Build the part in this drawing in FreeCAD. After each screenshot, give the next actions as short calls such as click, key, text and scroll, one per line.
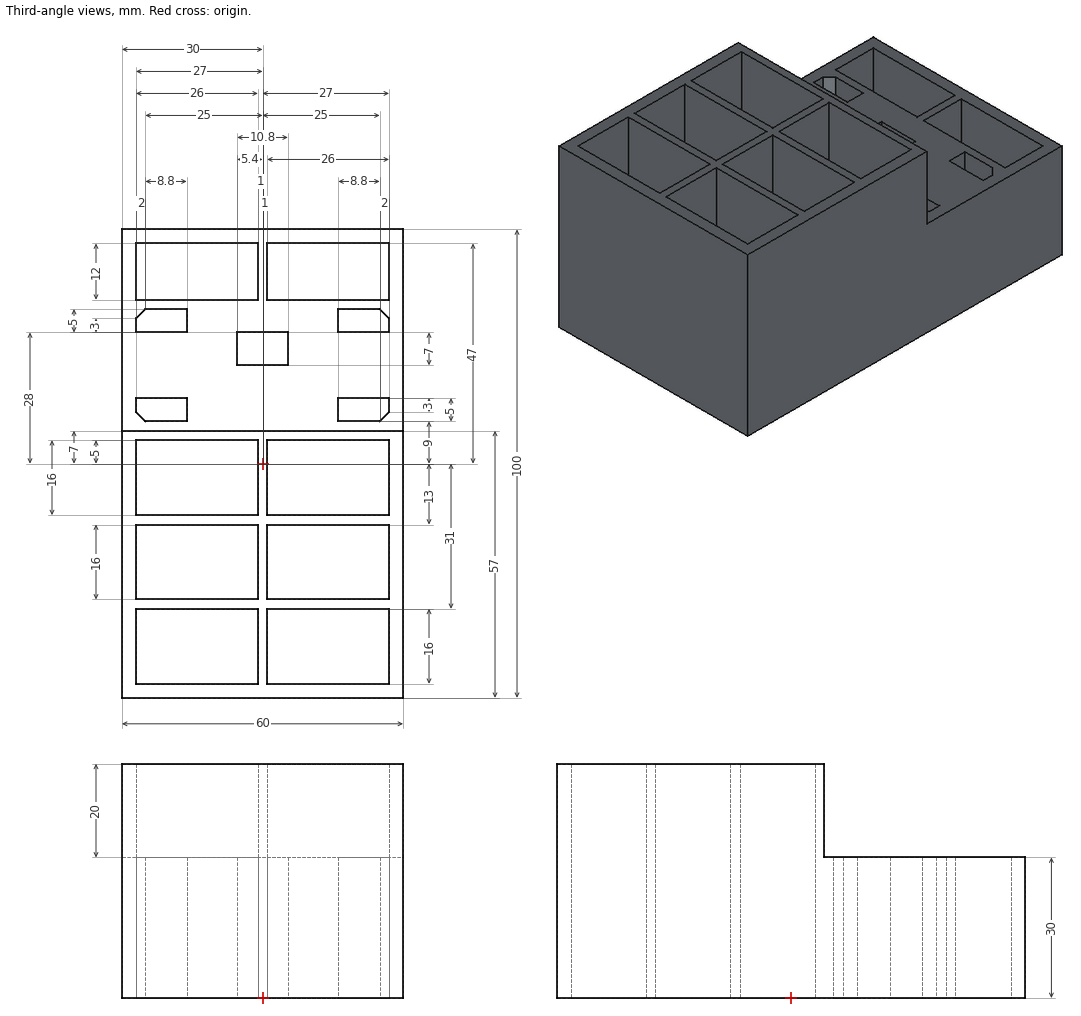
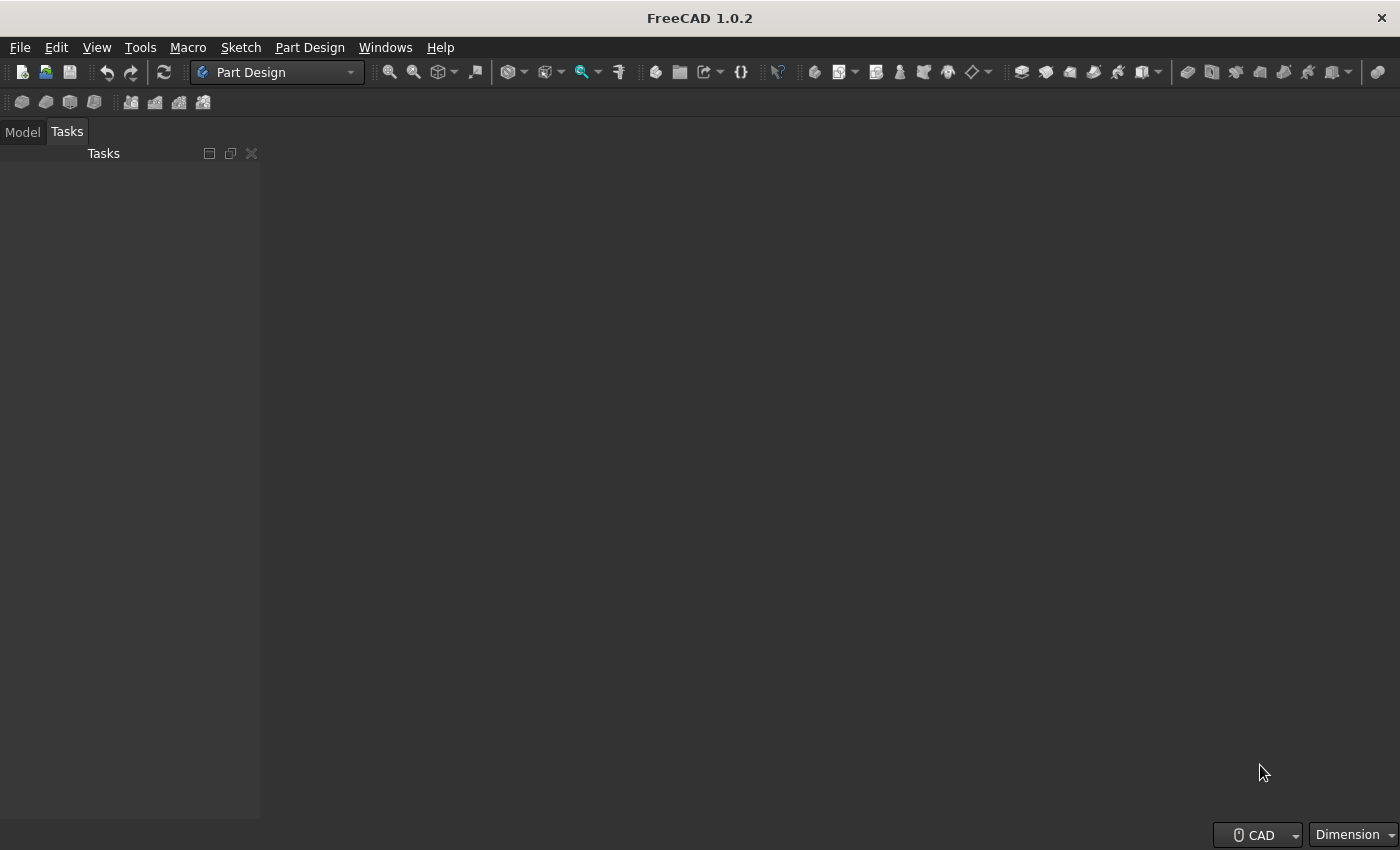
key(ctrl+n)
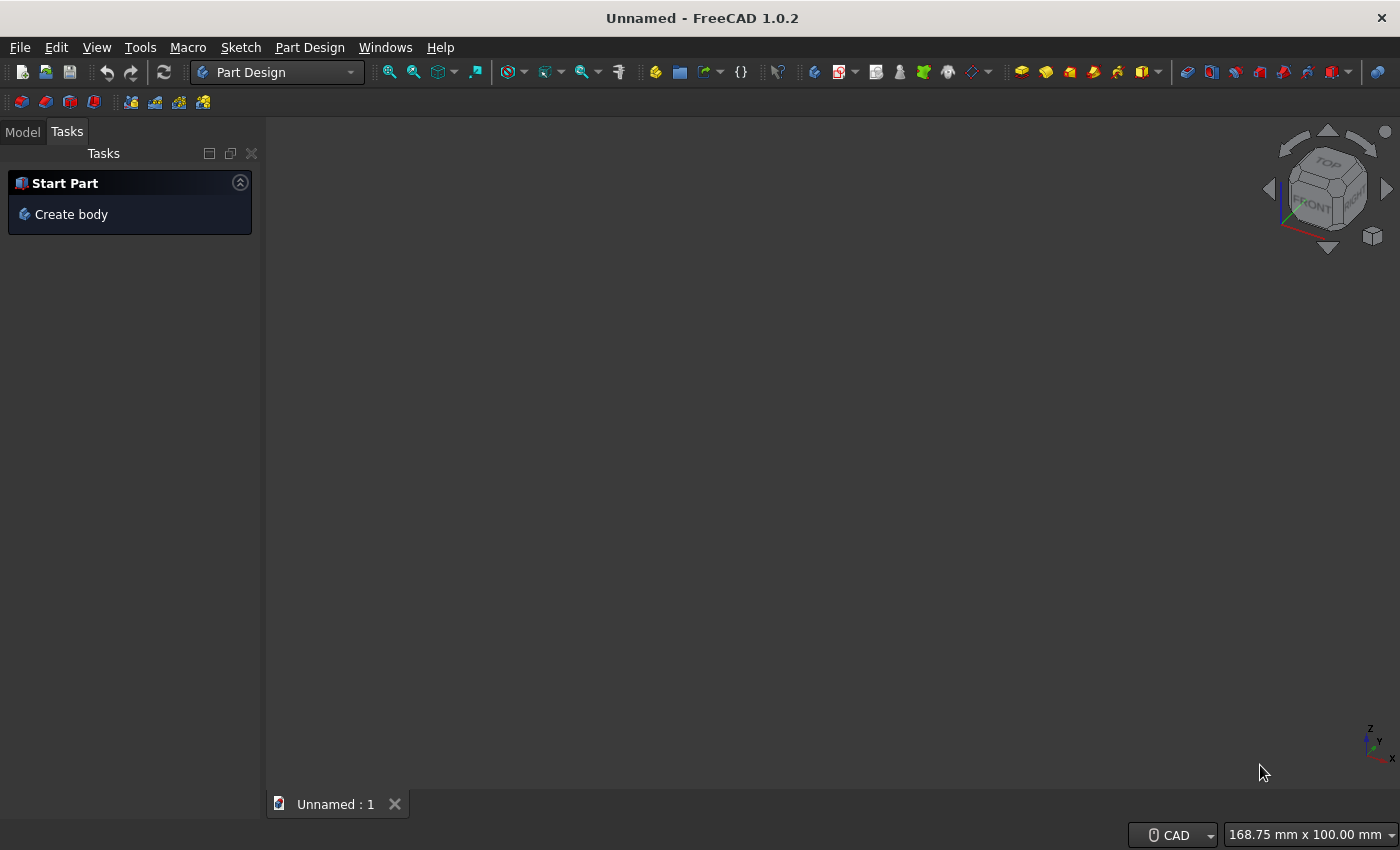
click(840, 72)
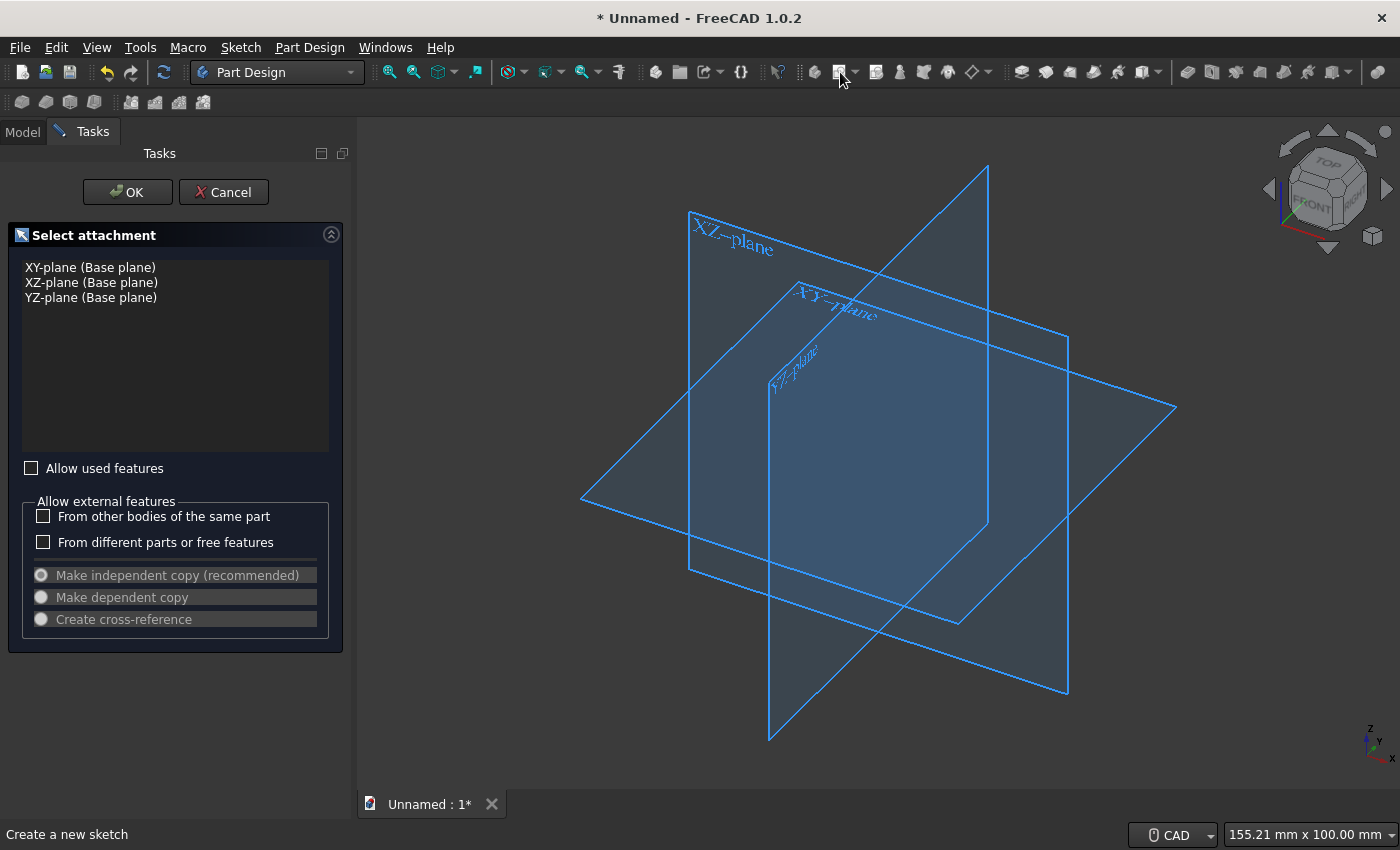
click(82, 268)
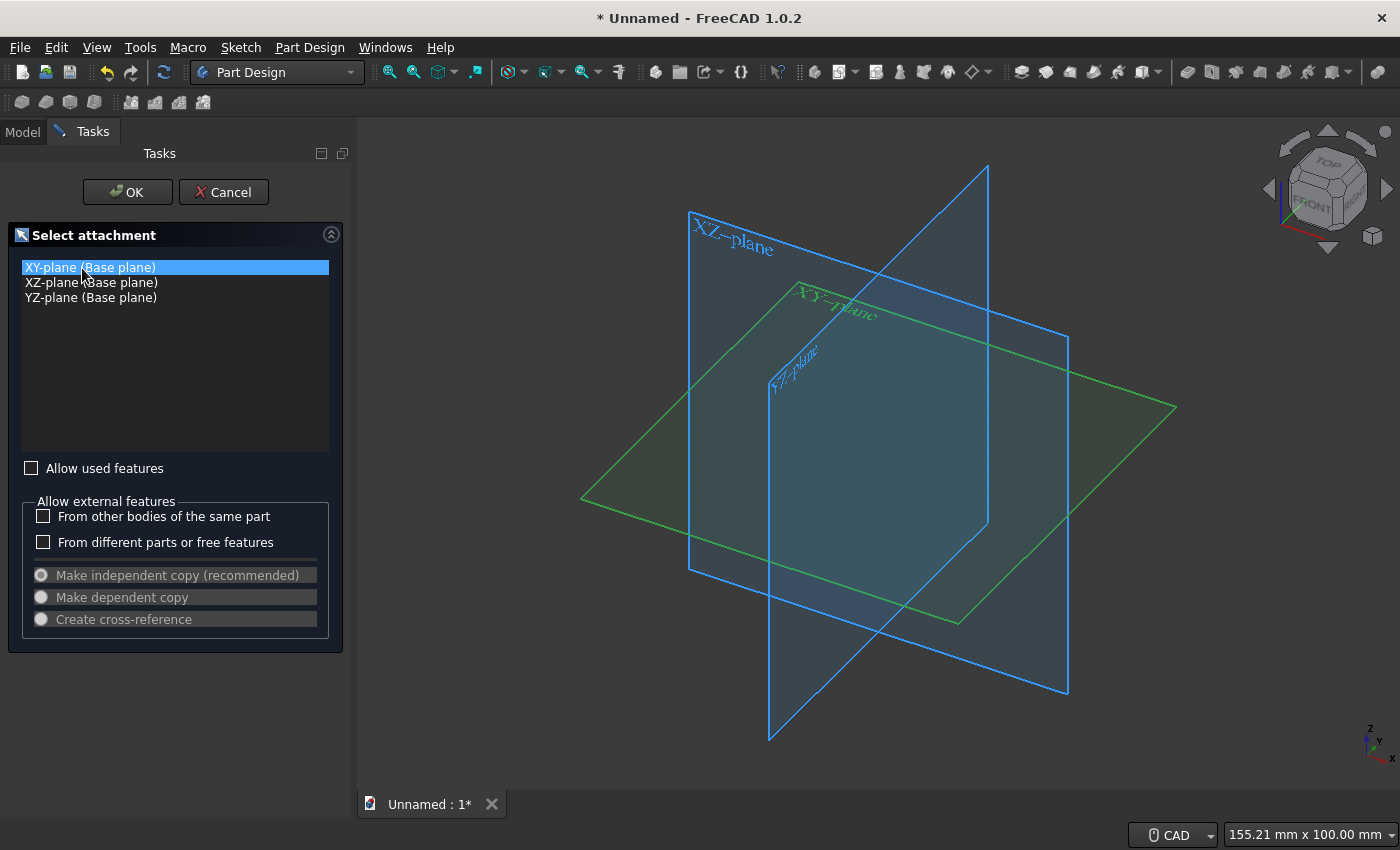
click(128, 192)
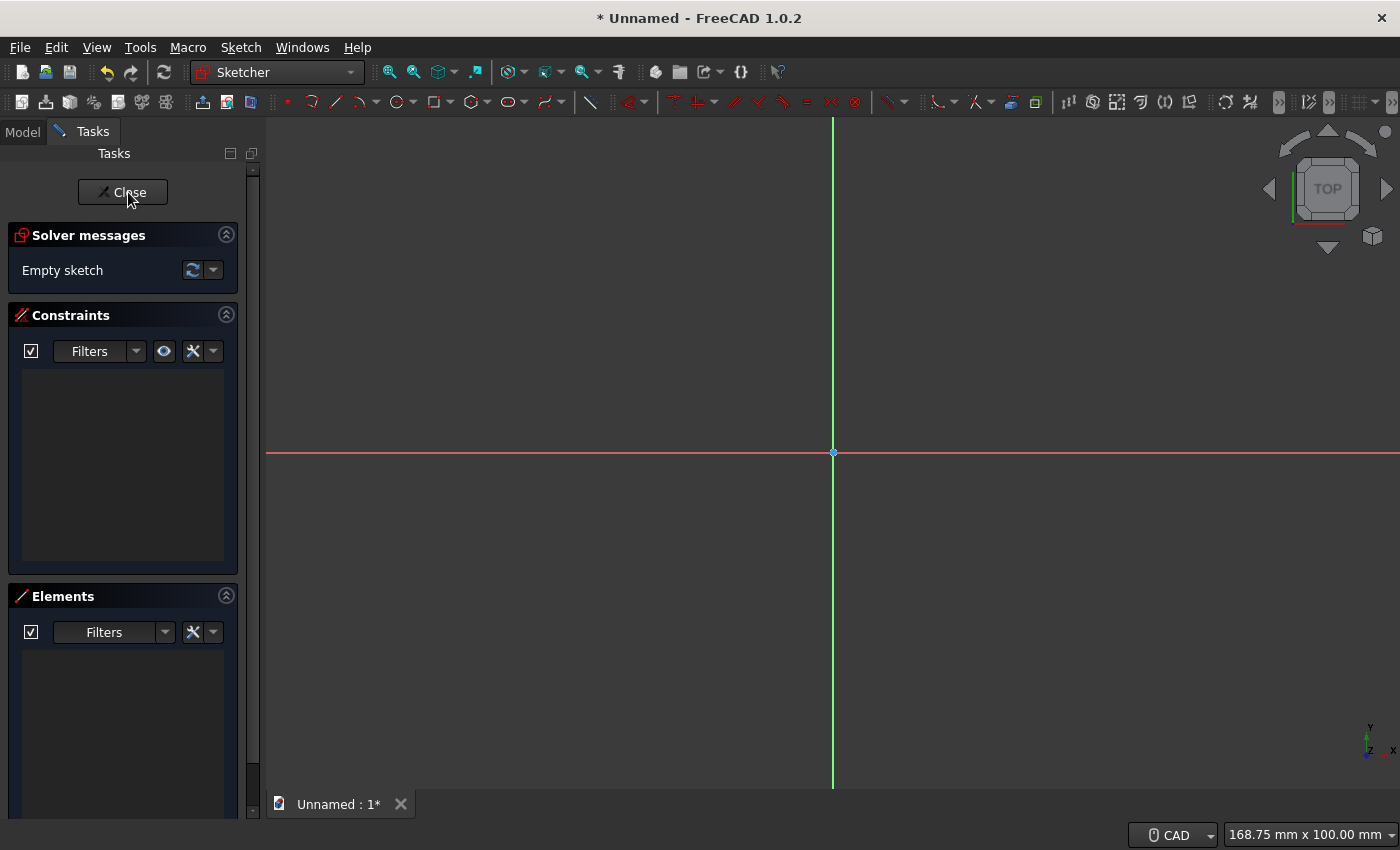
scroll(625, 453, down, 2)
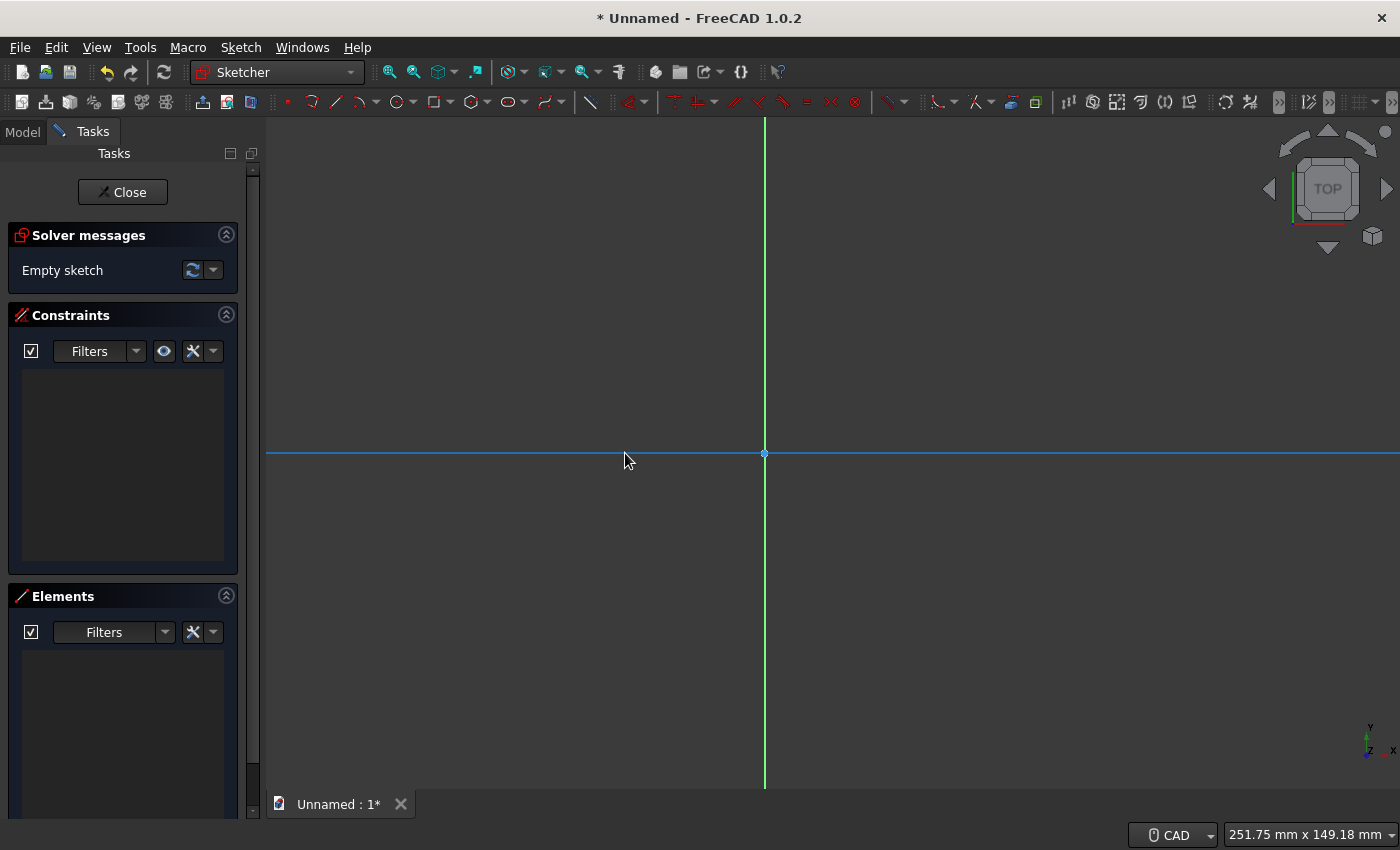
key(g)
key(v)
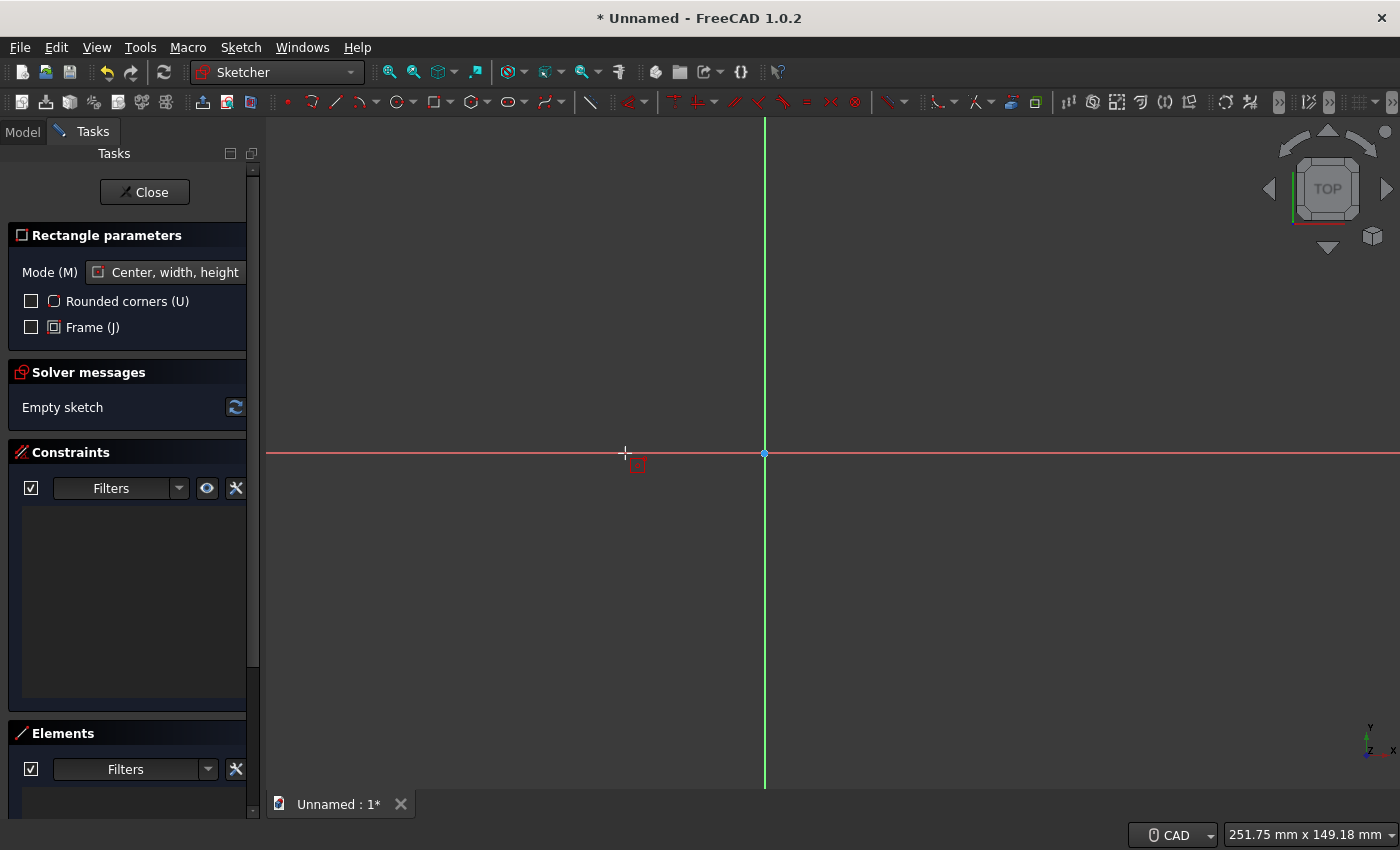
click(765, 453)
move(900, 228)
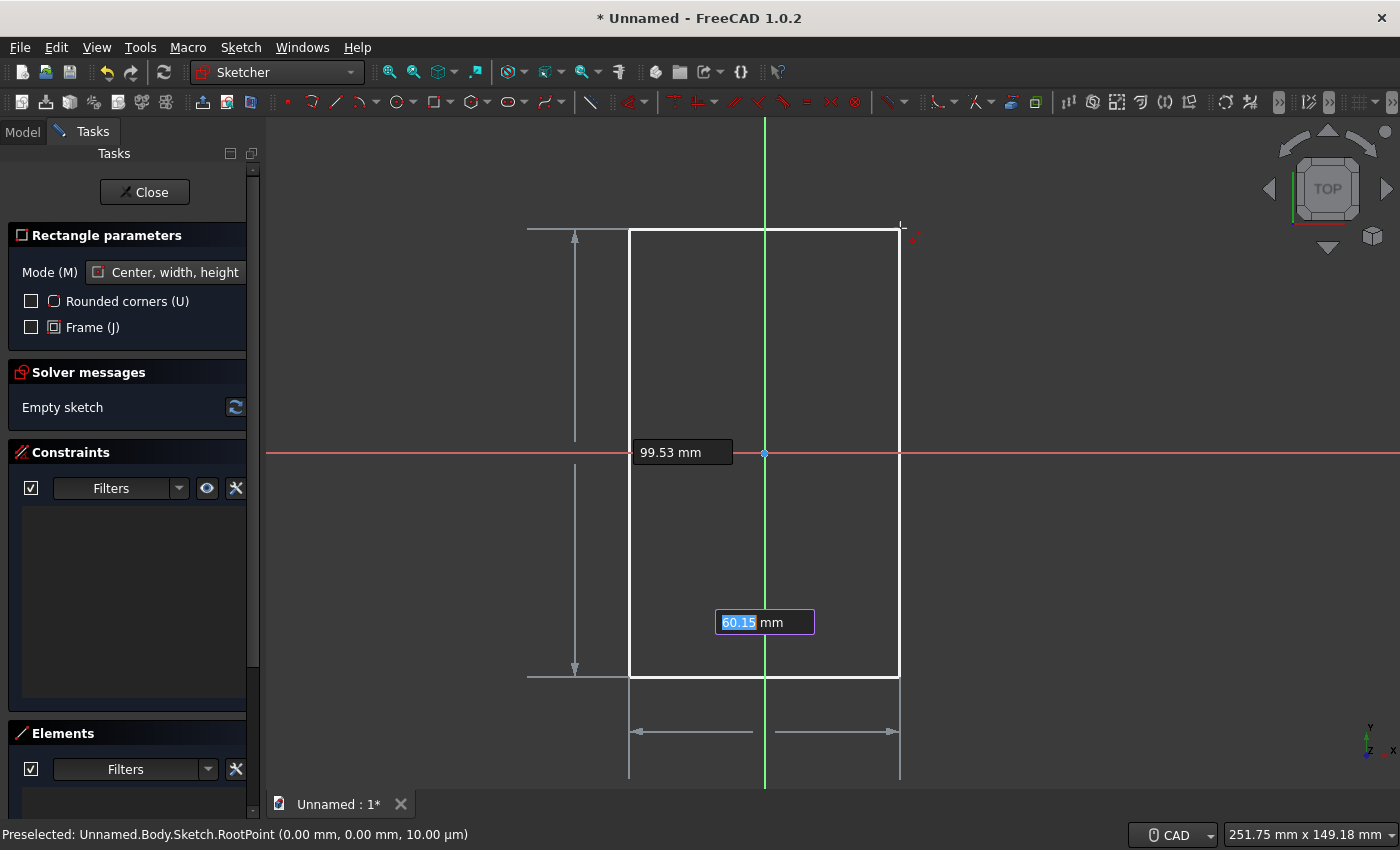
text(60)
key(Tab)
text(100)
key(Return)
key(Escape)